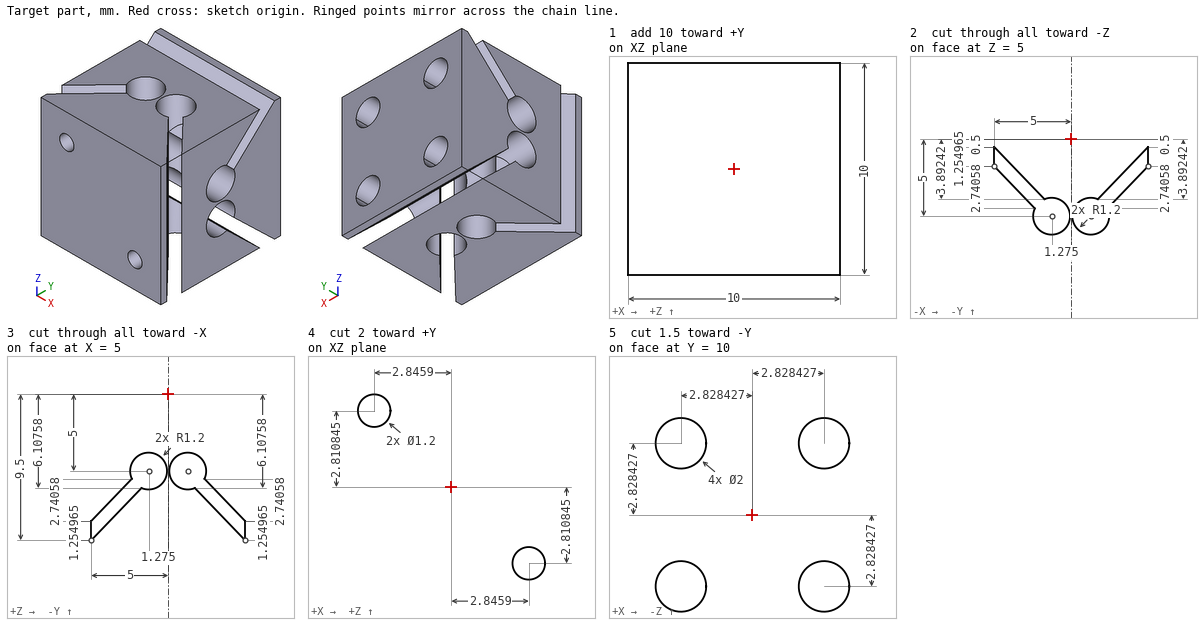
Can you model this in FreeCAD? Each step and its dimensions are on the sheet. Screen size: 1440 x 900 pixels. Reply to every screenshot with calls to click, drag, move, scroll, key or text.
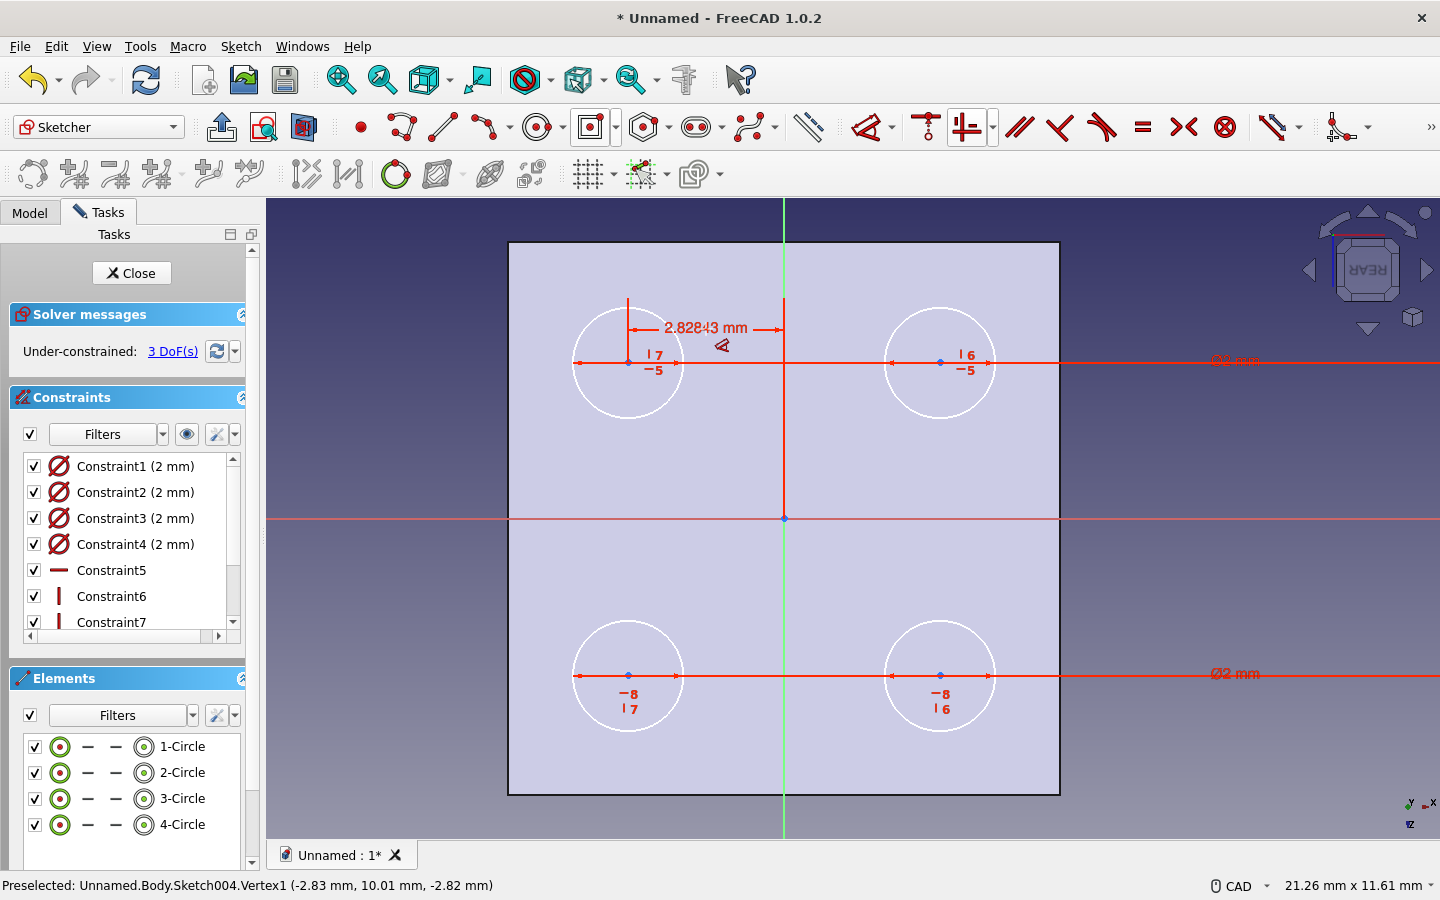
click(628, 363)
click(594, 441)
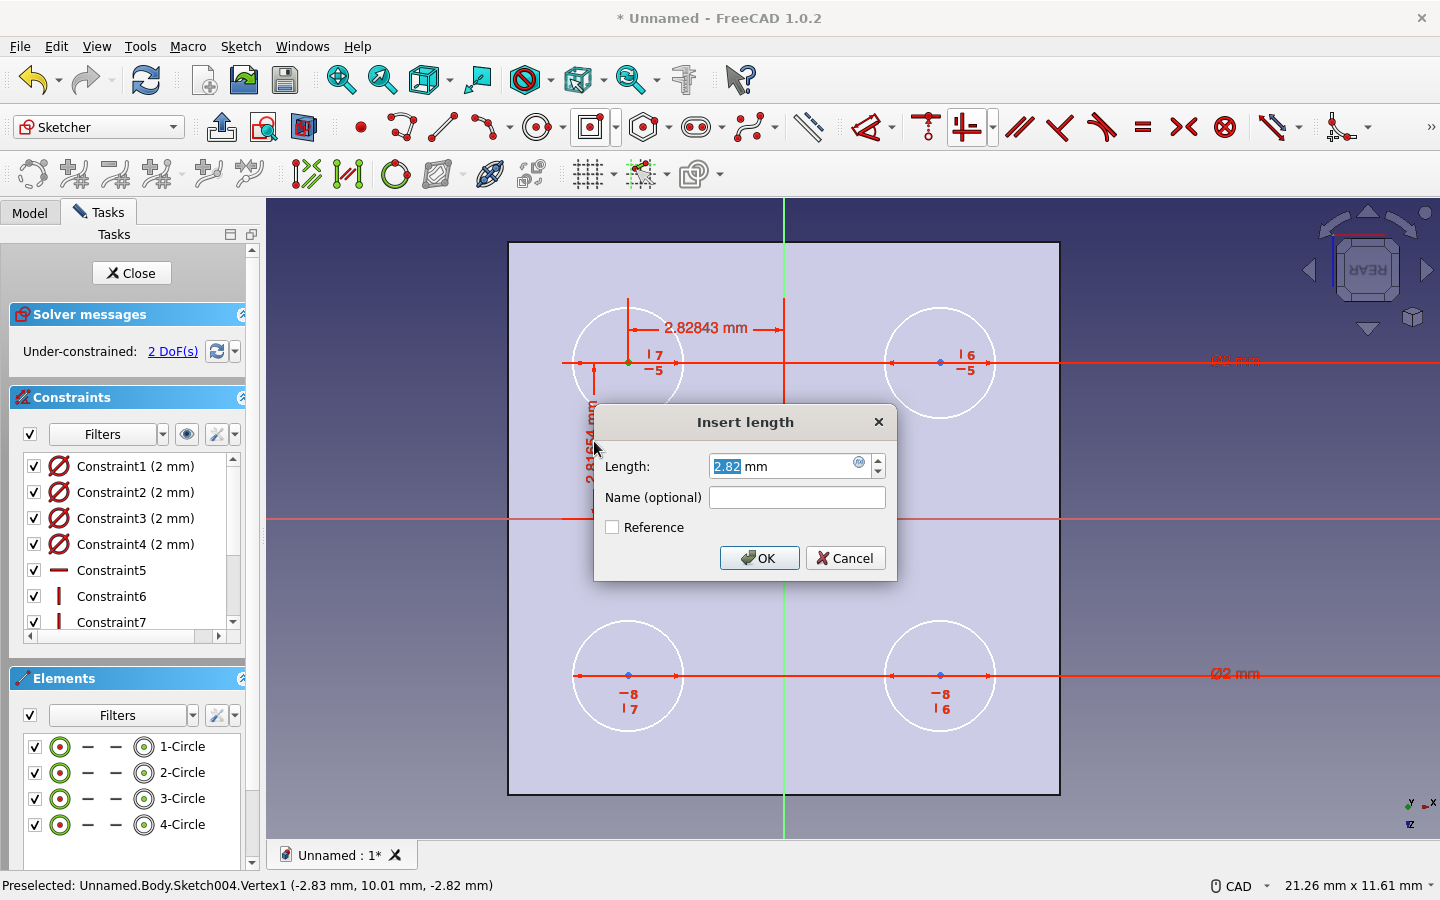
text(2.828427)
key(Return)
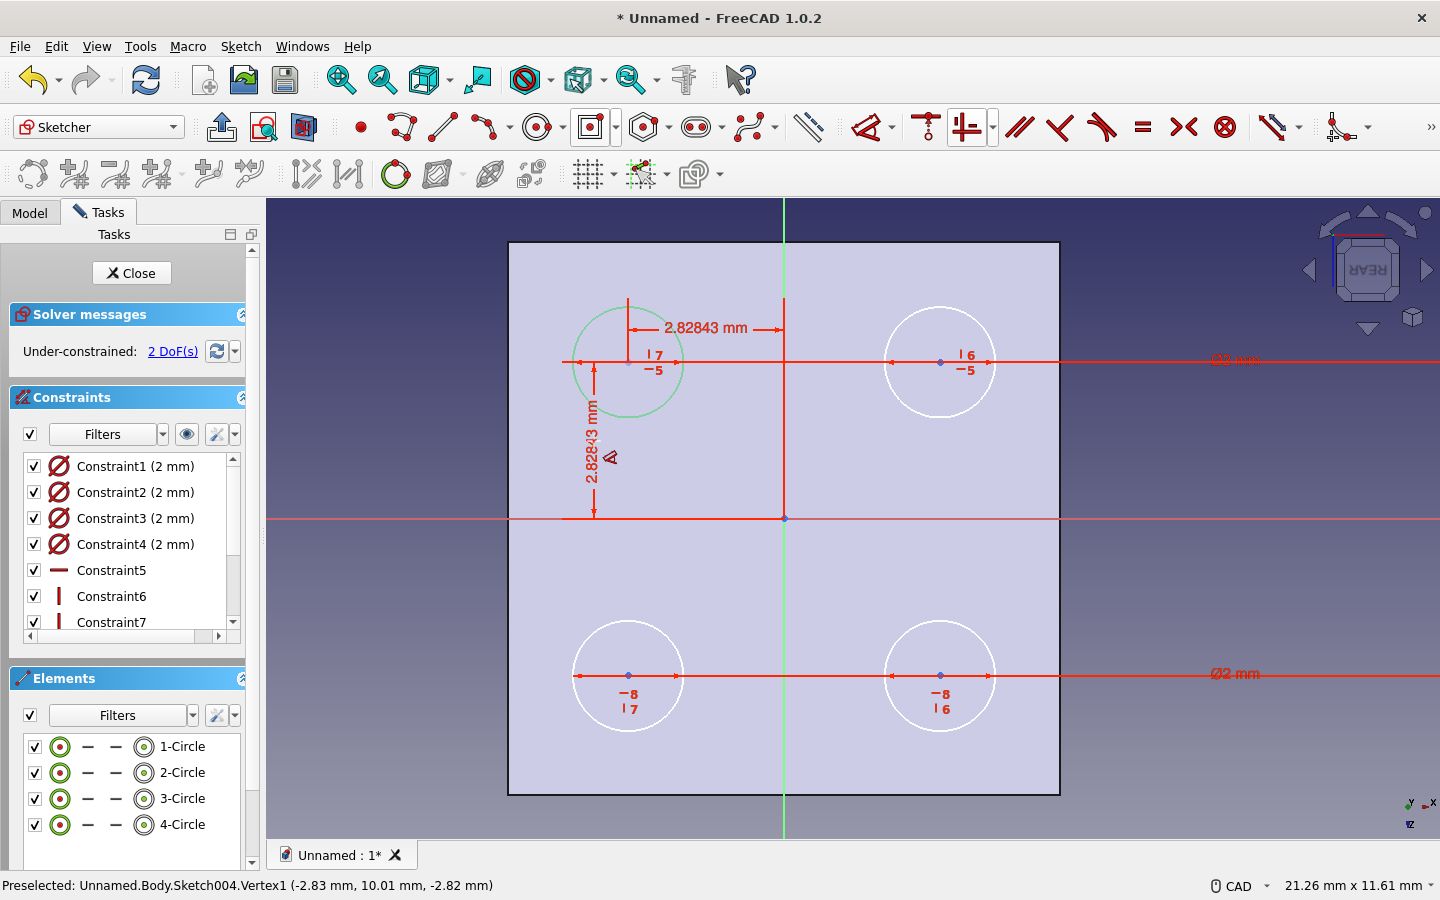
click(940, 362)
click(862, 328)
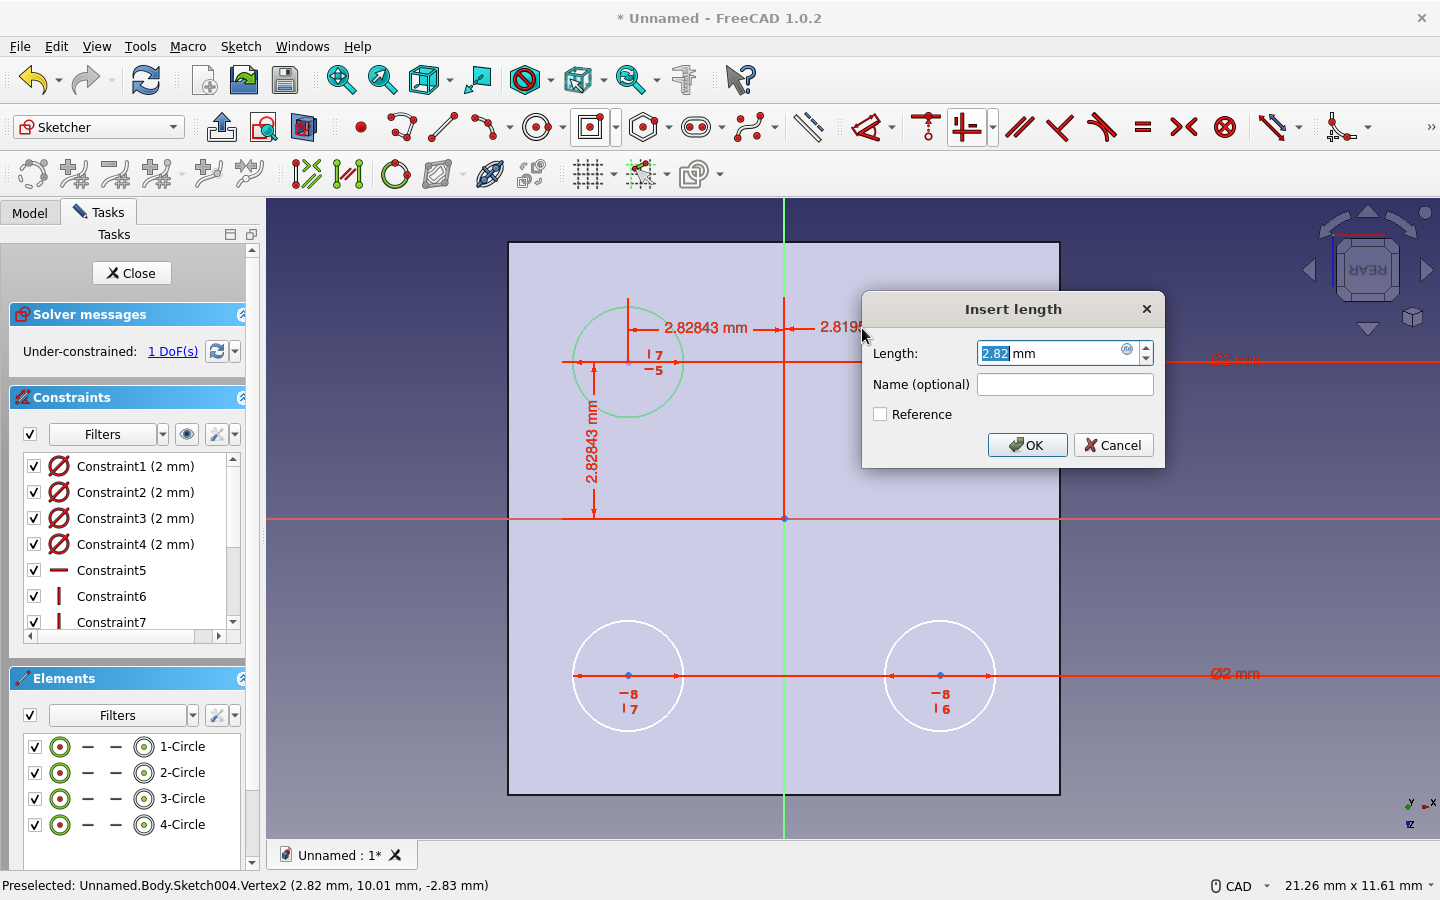
text(2.828427)
key(Return)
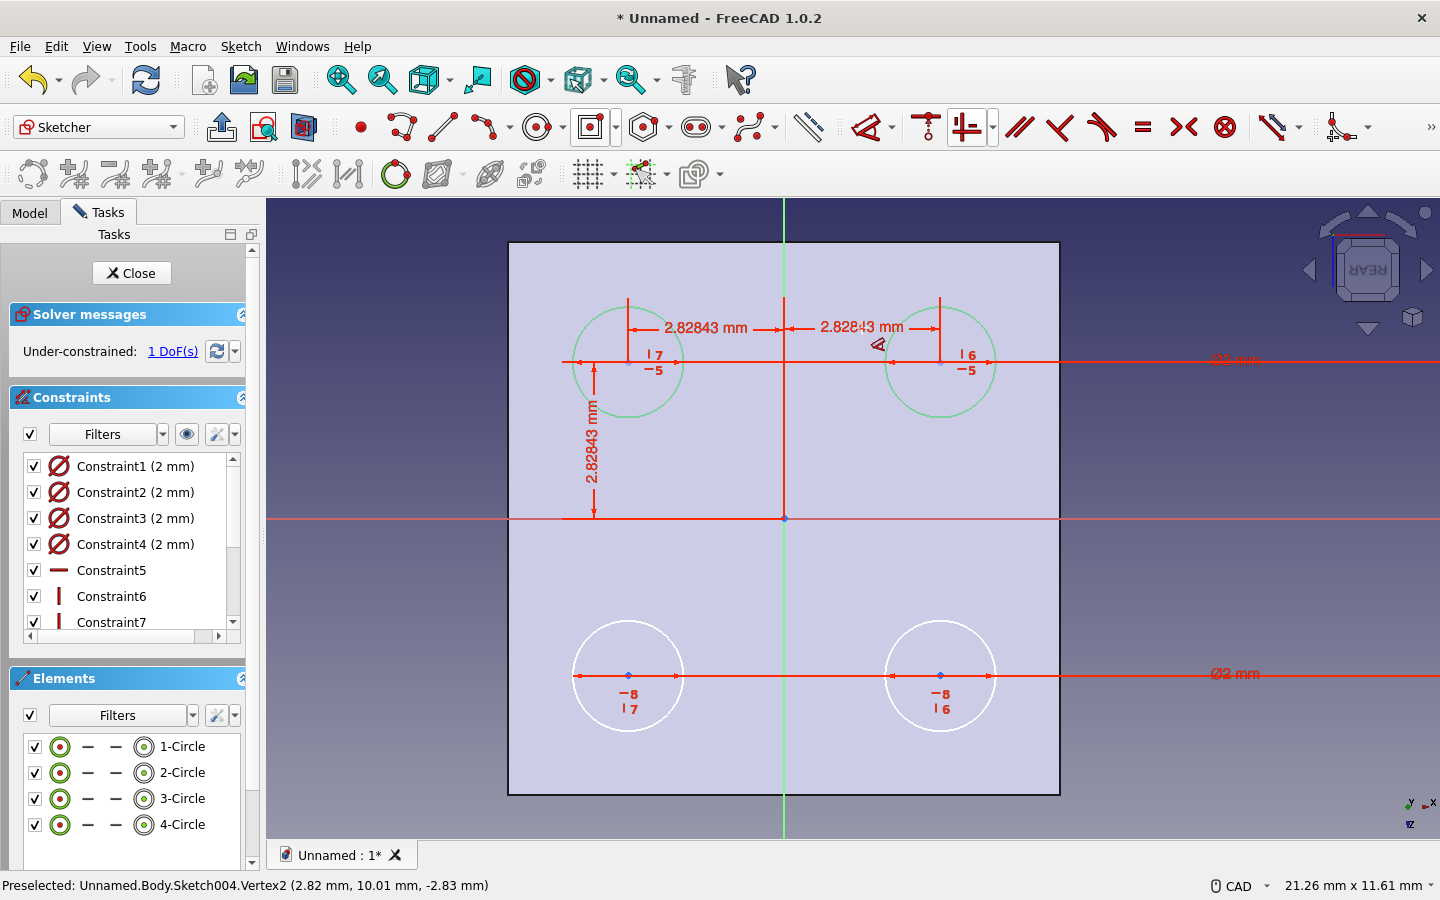
click(940, 676)
click(974, 597)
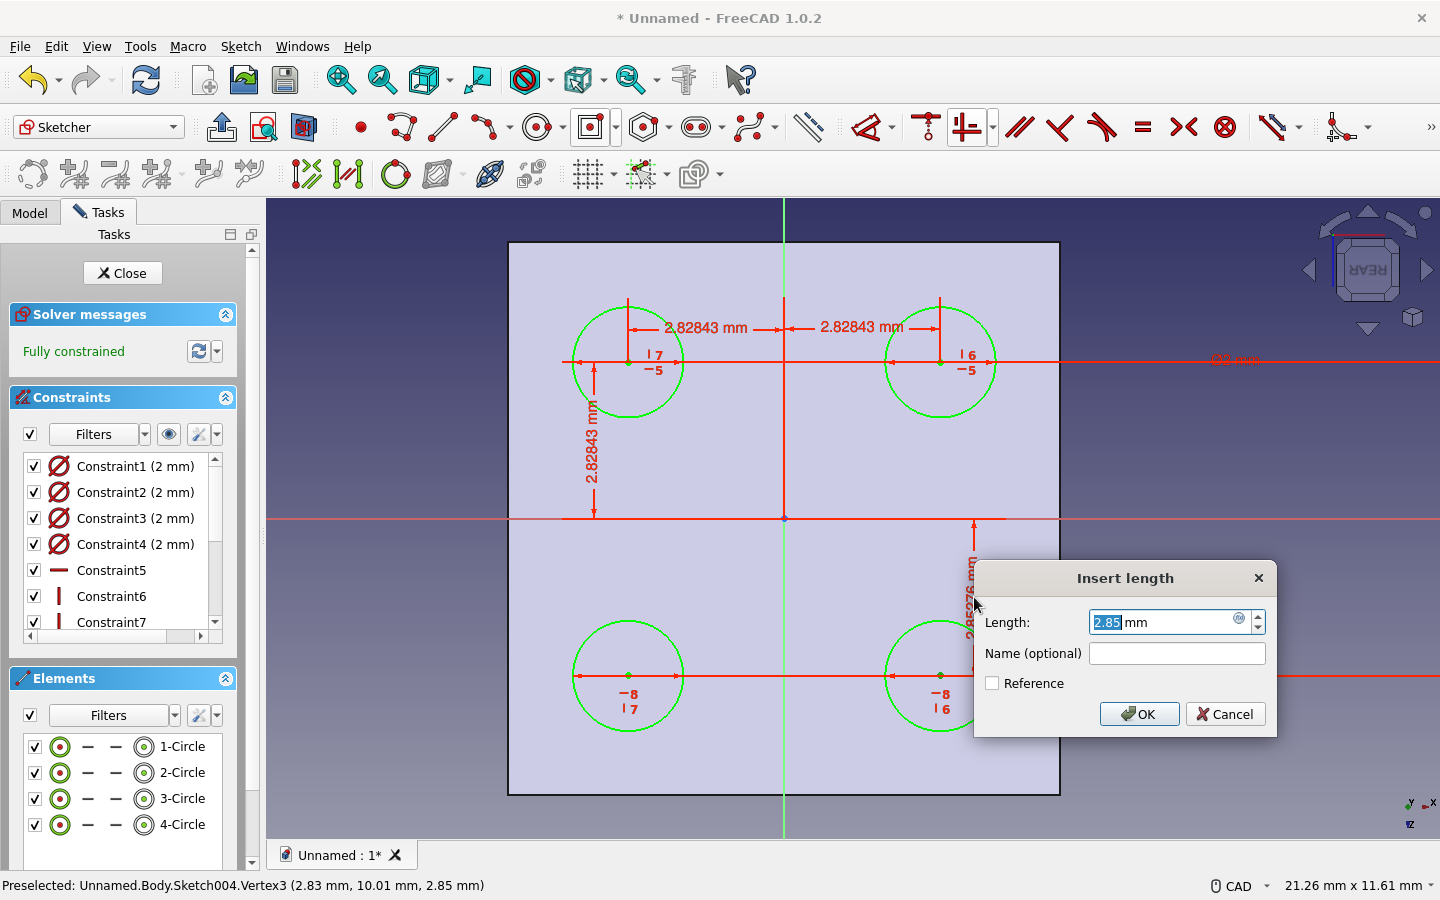
text(2.828427)
key(Return)
key(Escape)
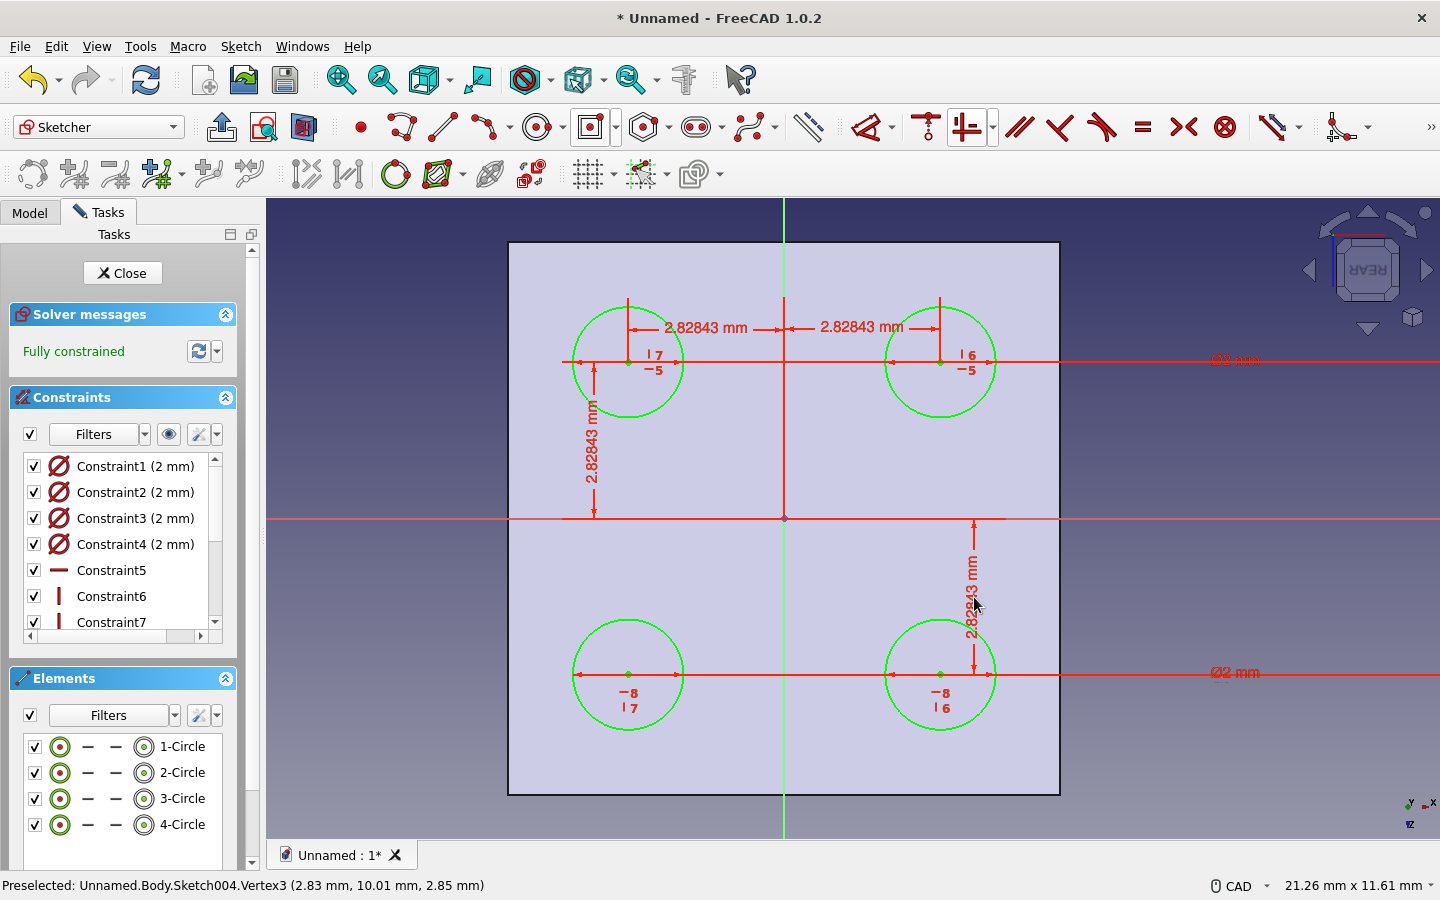
click(123, 273)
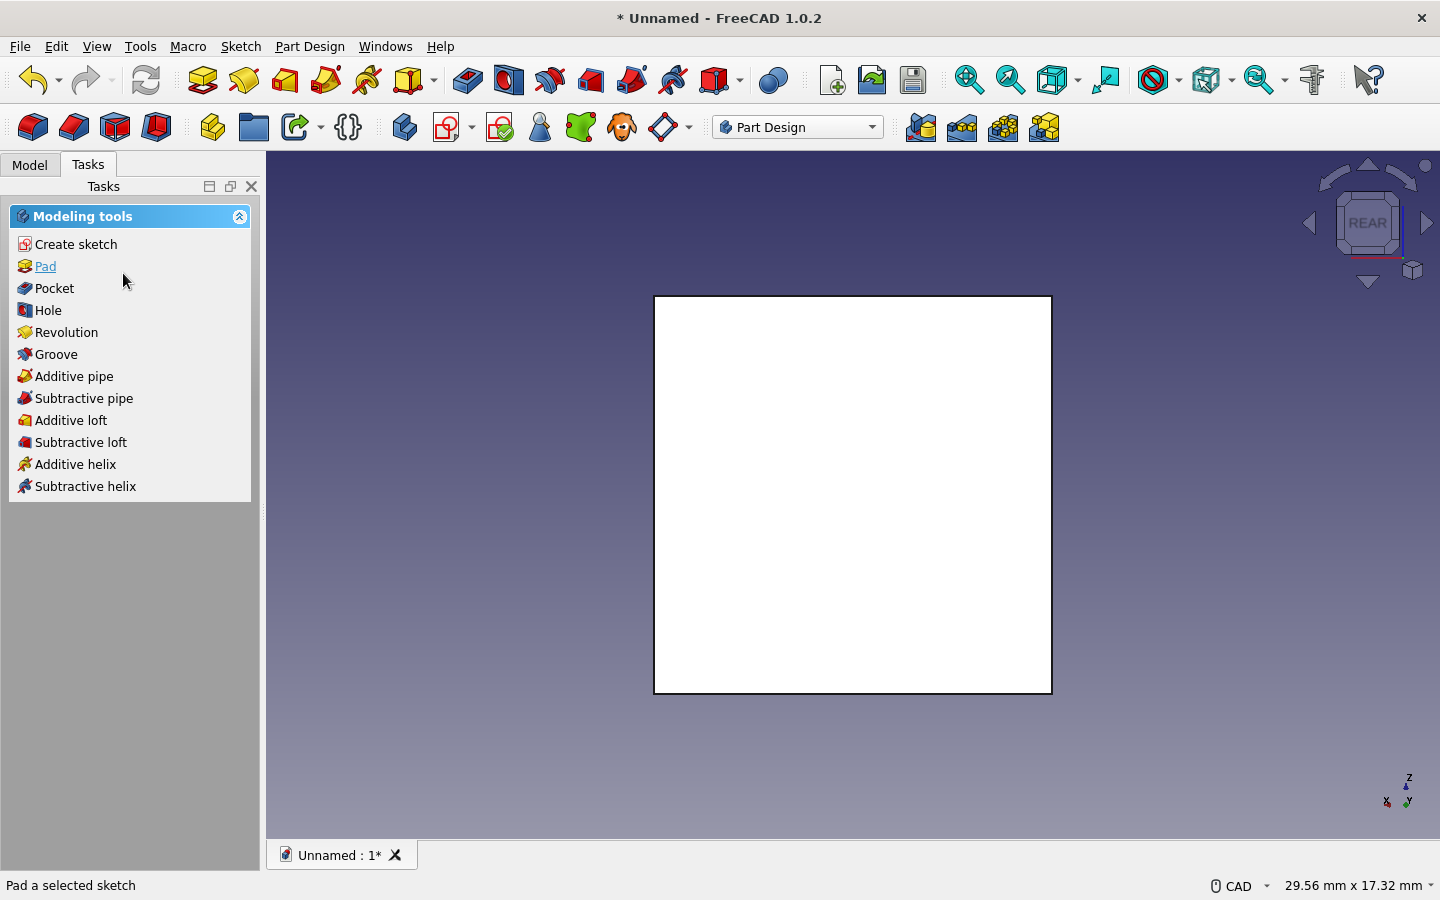
click(468, 80)